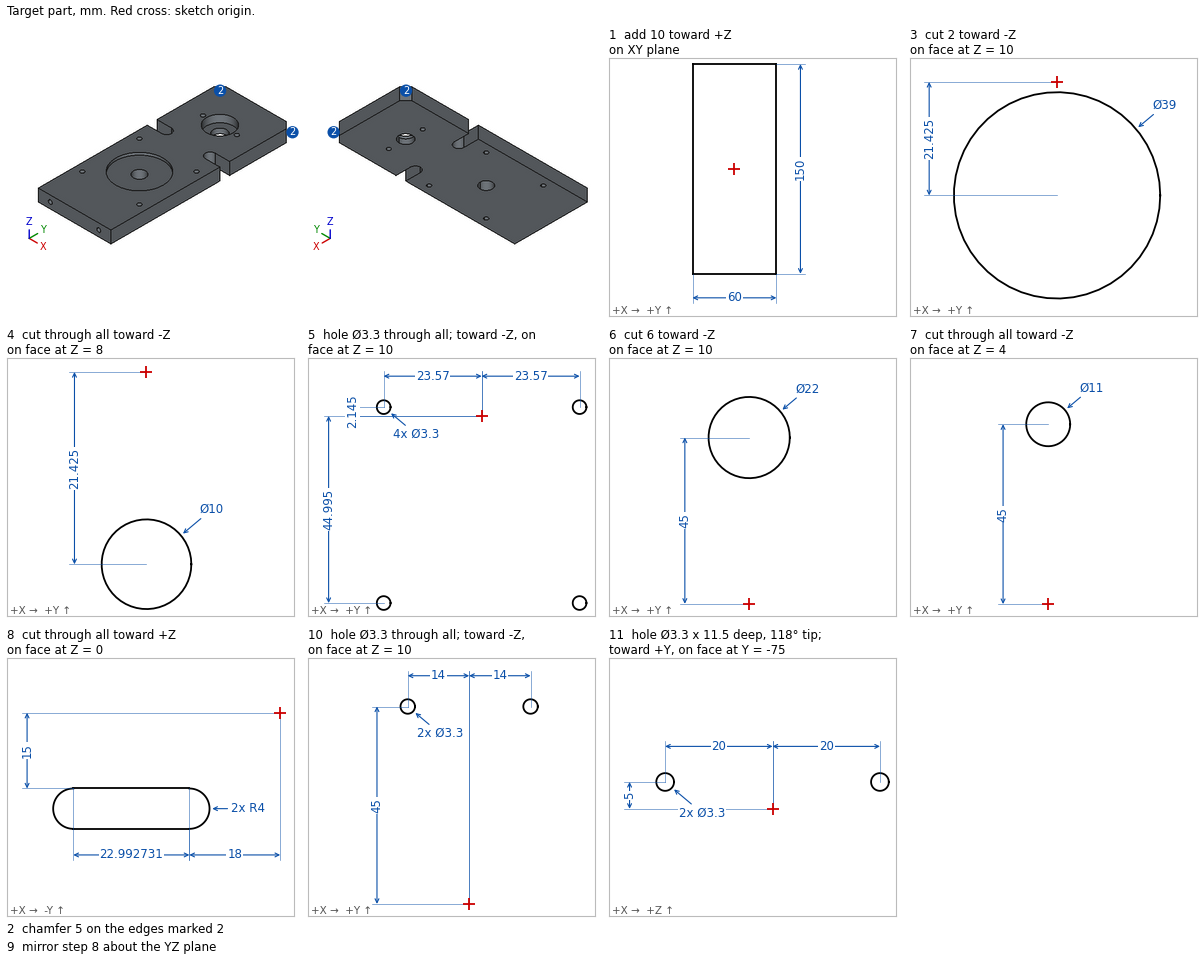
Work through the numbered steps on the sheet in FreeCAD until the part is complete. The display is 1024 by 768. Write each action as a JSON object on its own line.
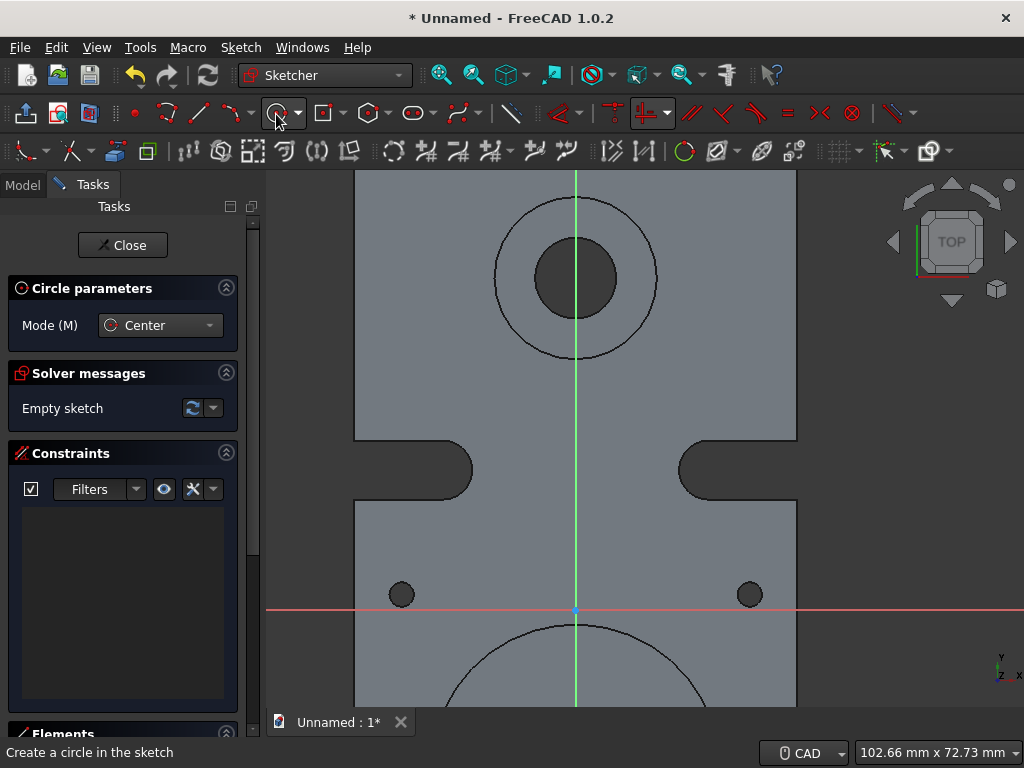
{"action": "scroll", "coordinate": [472, 278], "scroll_direction": "up", "scroll_amount": 4}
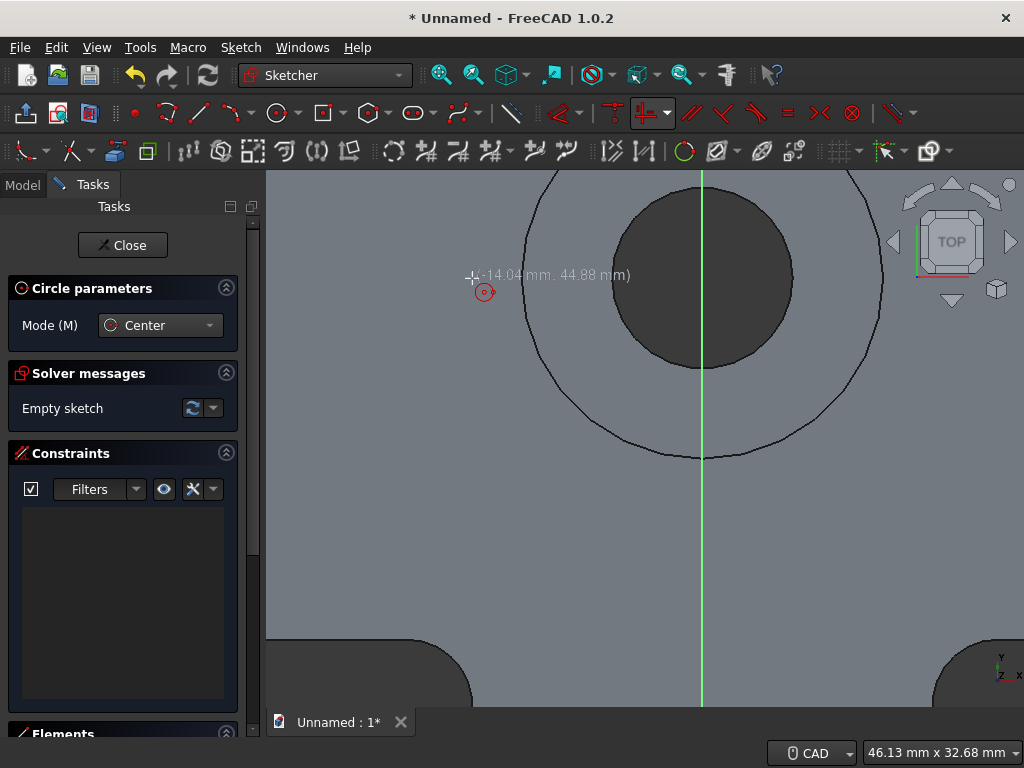
{"action": "left_click", "coordinate": [472, 278]}
{"action": "left_click", "coordinate": [491, 259]}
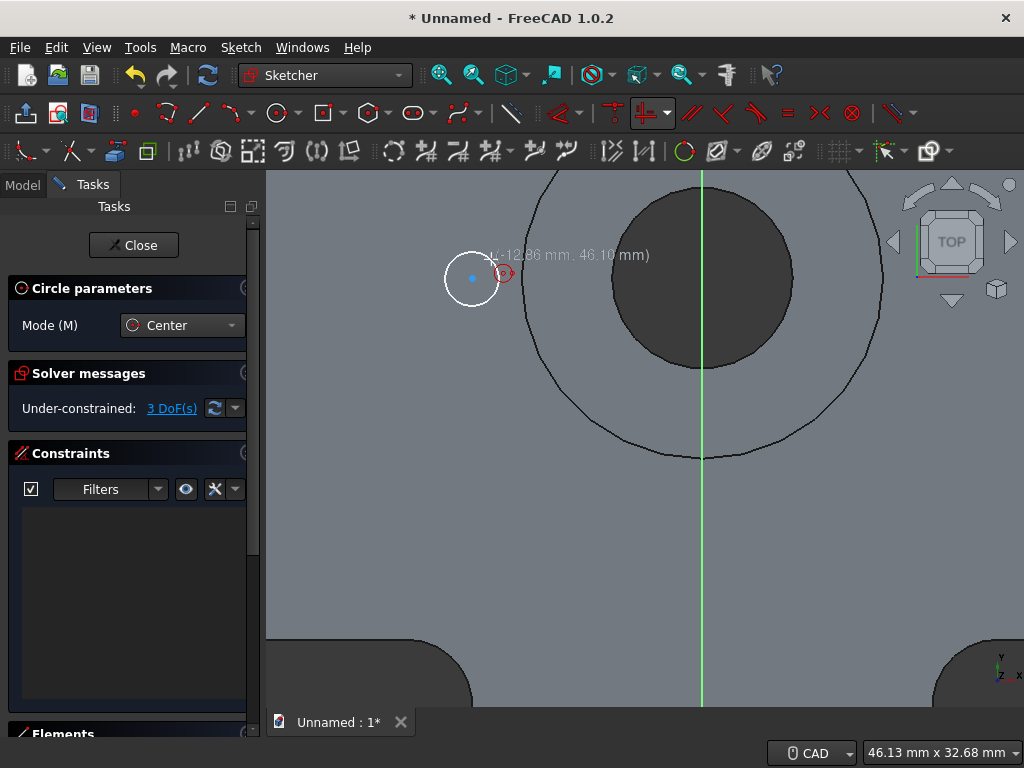
{"action": "scroll", "coordinate": [474, 279], "scroll_direction": "down", "scroll_amount": 4}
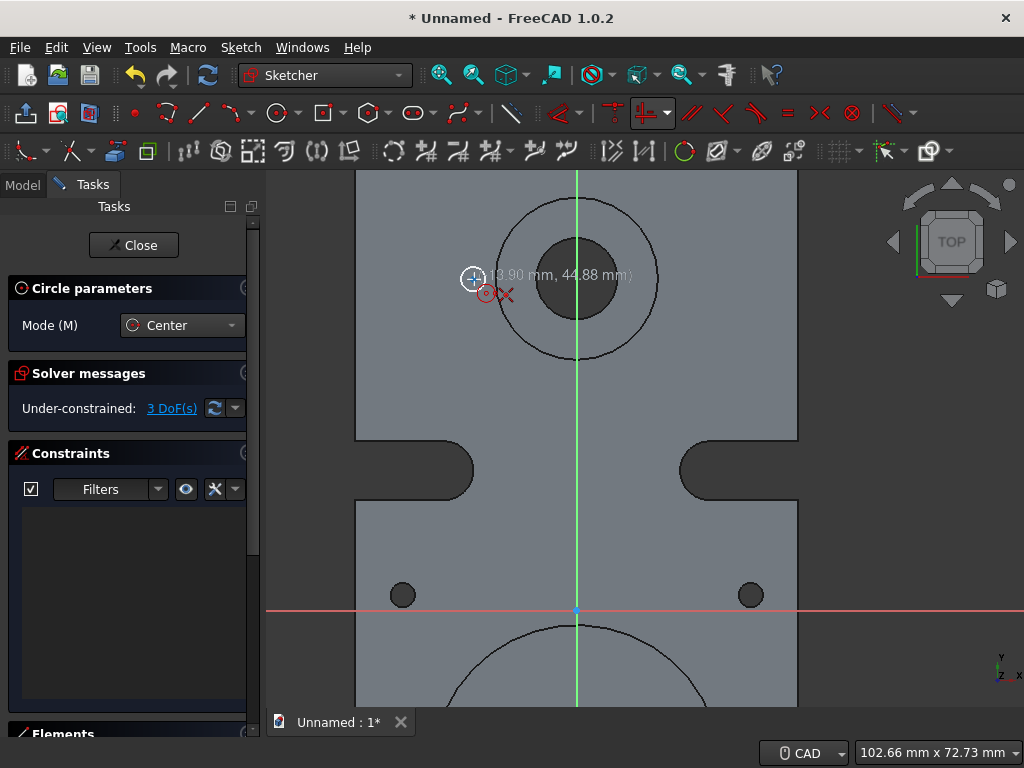
{"action": "scroll", "coordinate": [680, 279], "scroll_direction": "up", "scroll_amount": 4}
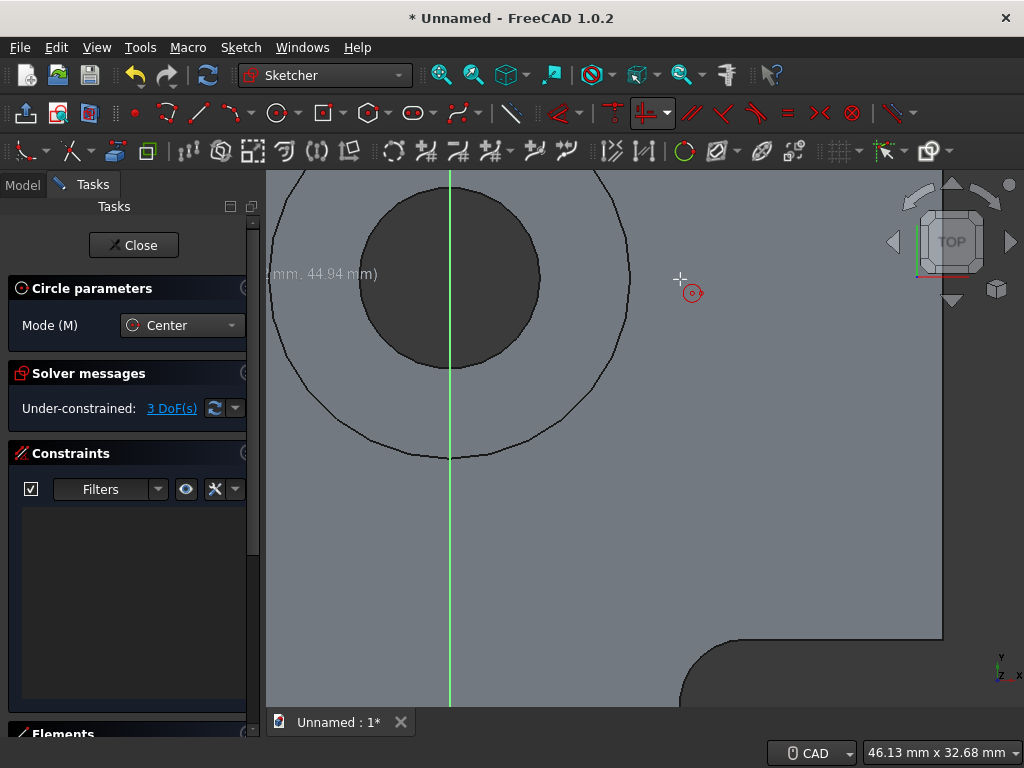
{"action": "left_click", "coordinate": [680, 278]}
{"action": "left_click", "coordinate": [699, 259]}
{"action": "key", "text": "Escape"}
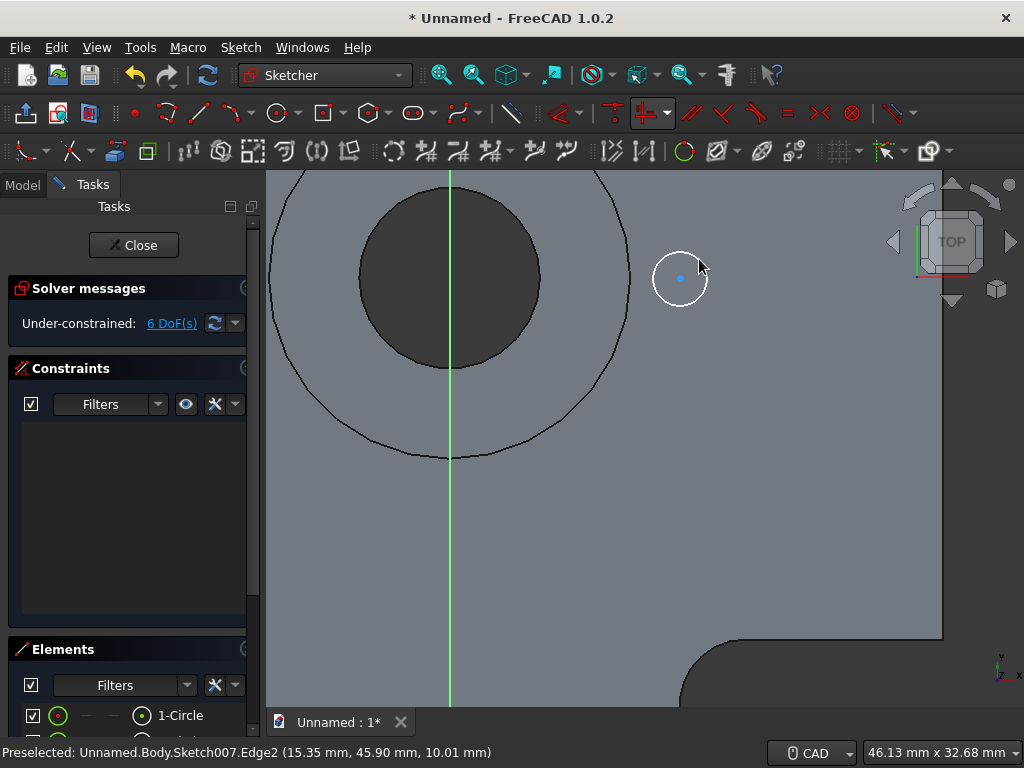
{"action": "scroll", "coordinate": [680, 279], "scroll_direction": "down", "scroll_amount": 4}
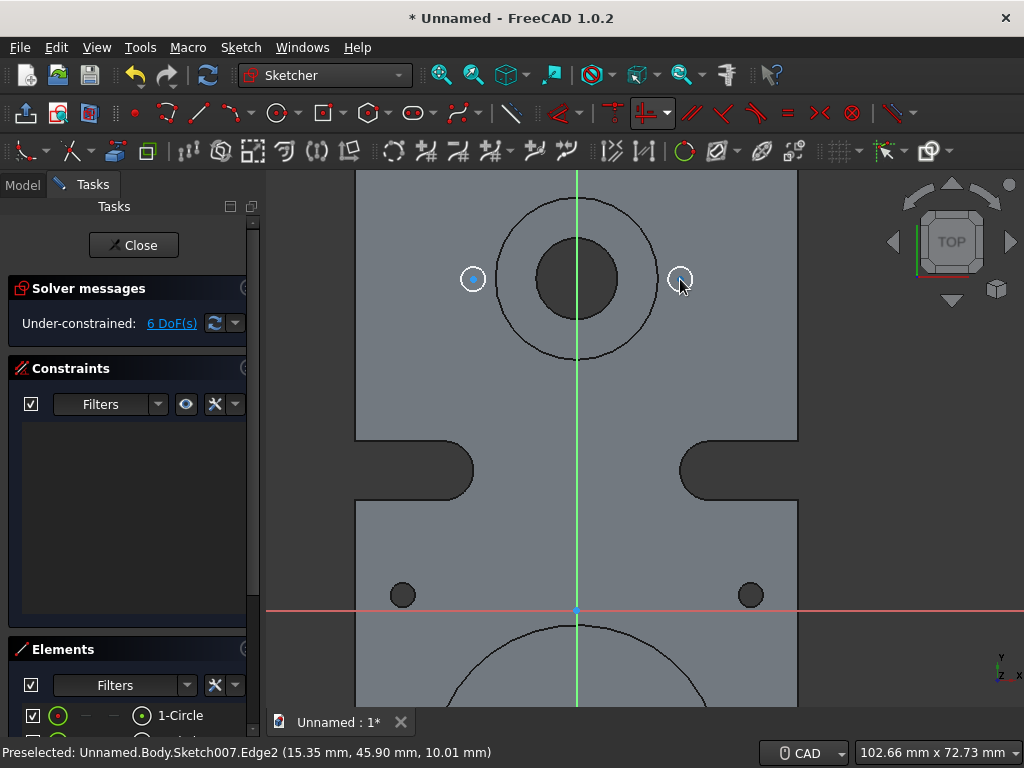
{"action": "left_click", "coordinate": [482, 271]}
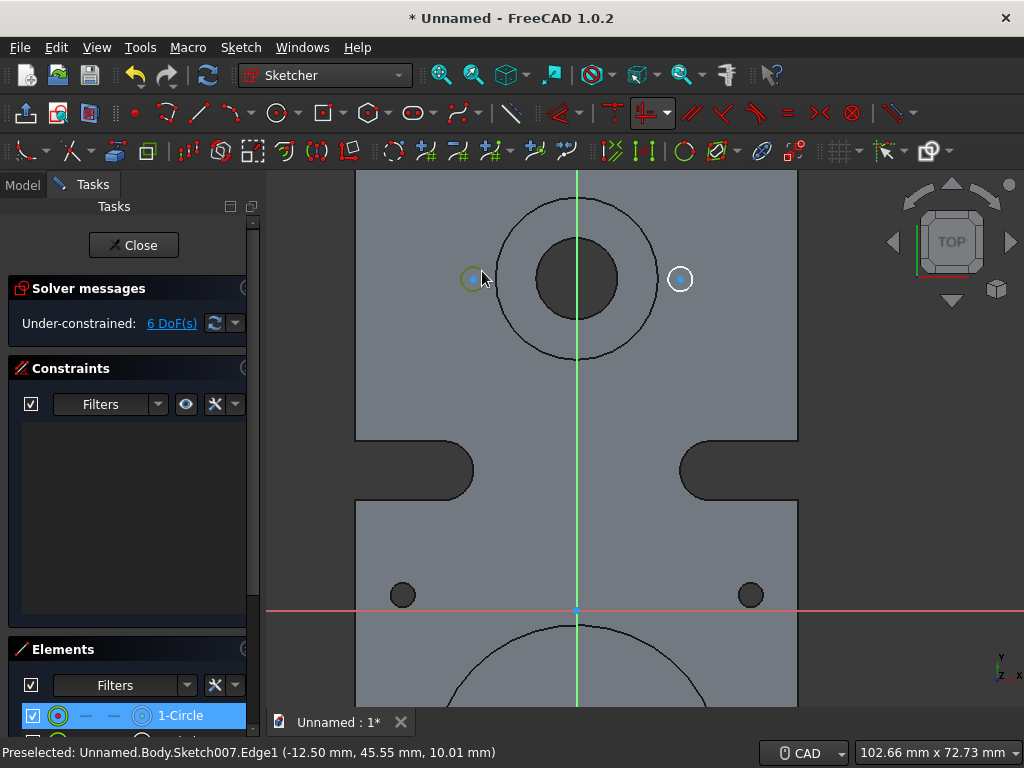
{"action": "left_click", "coordinate": [689, 271]}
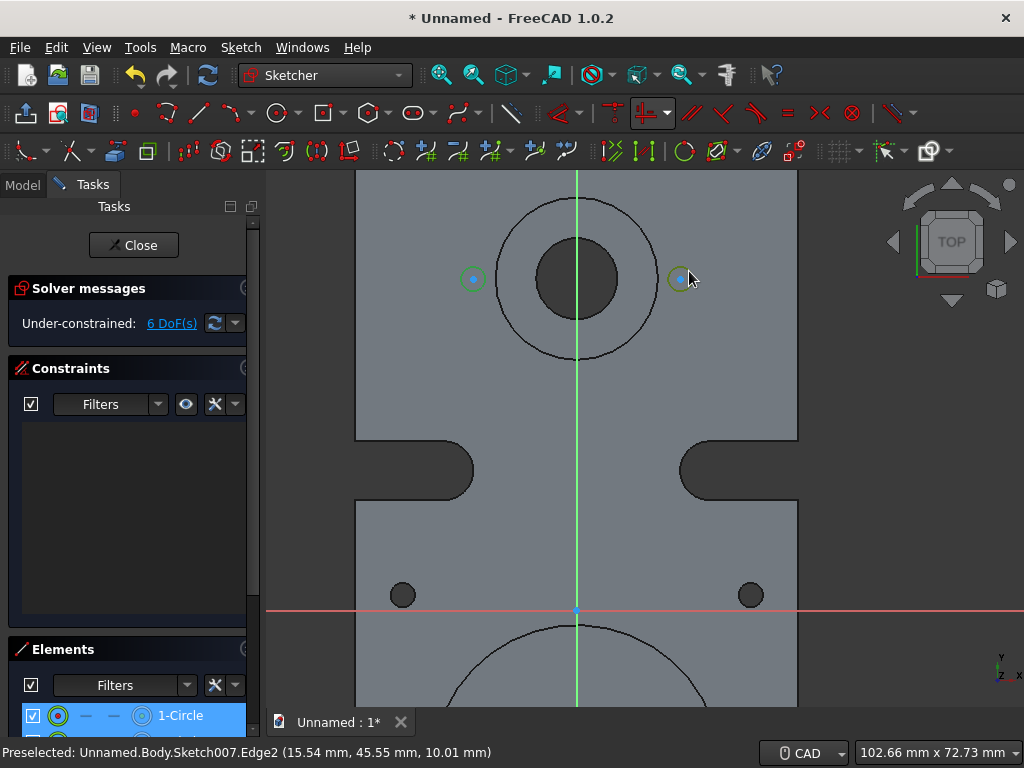
{"action": "left_click", "coordinate": [788, 114]}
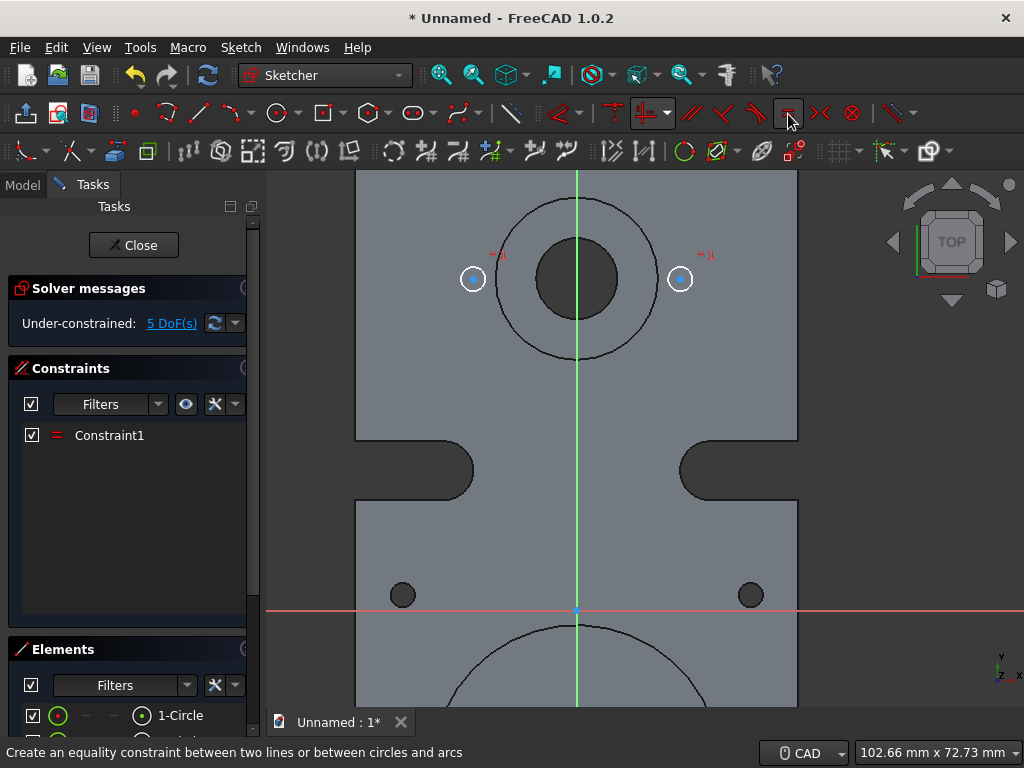
{"action": "left_click", "coordinate": [473, 279]}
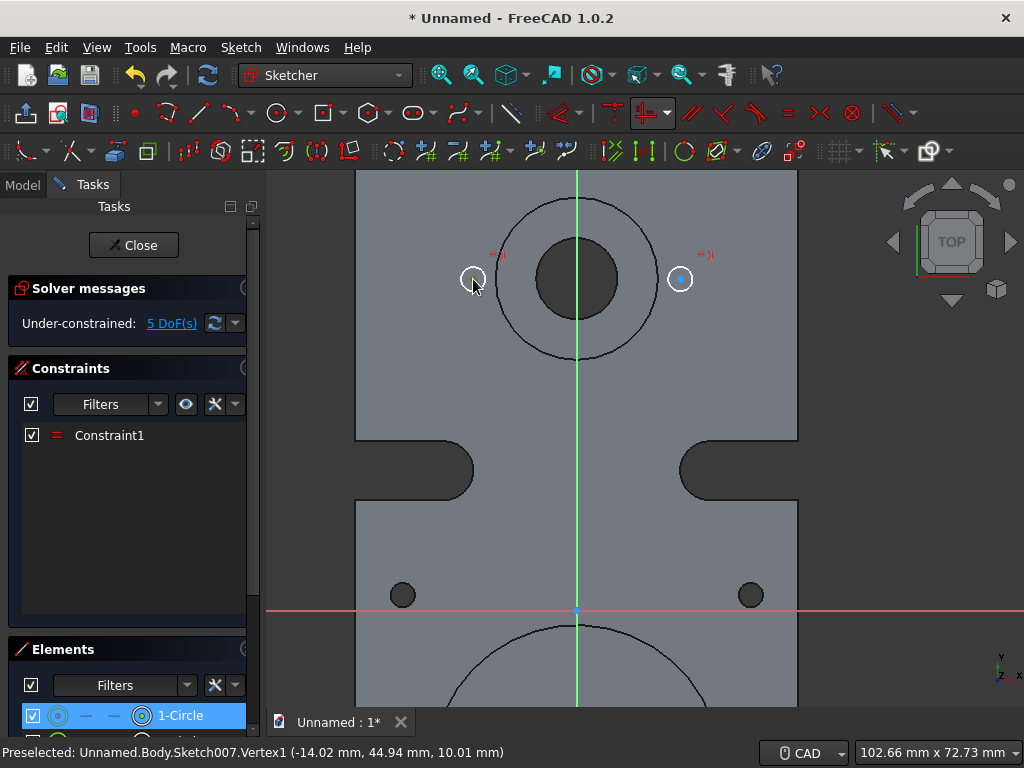
{"action": "left_click", "coordinate": [680, 279]}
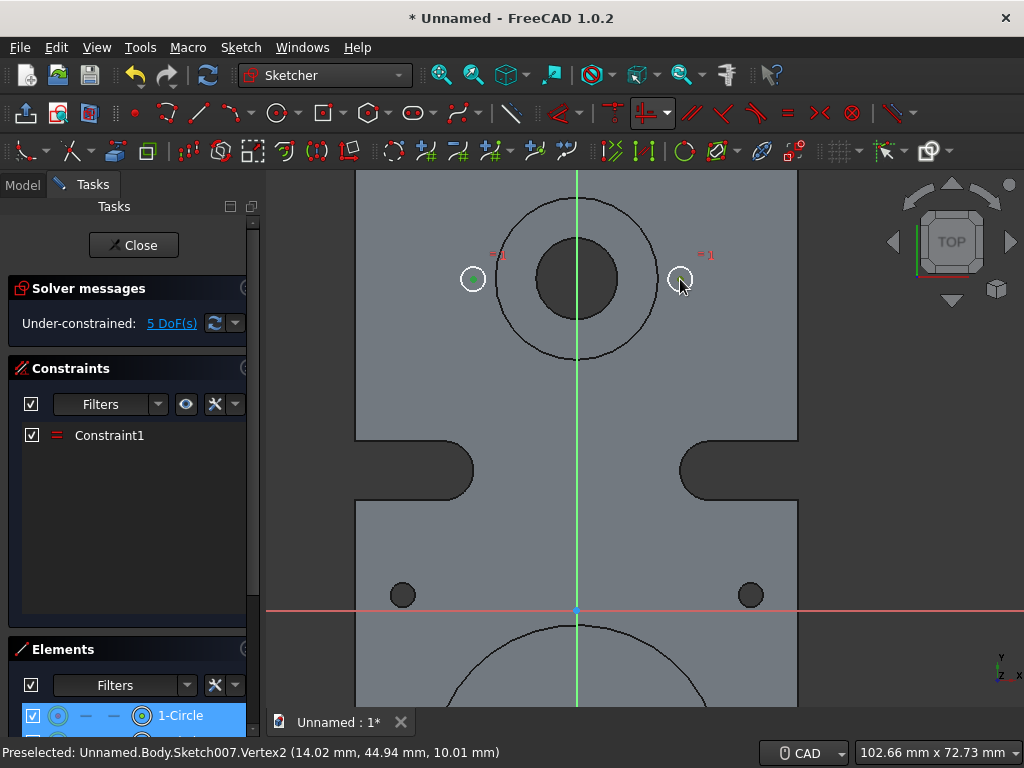
{"action": "left_click", "coordinate": [670, 114]}